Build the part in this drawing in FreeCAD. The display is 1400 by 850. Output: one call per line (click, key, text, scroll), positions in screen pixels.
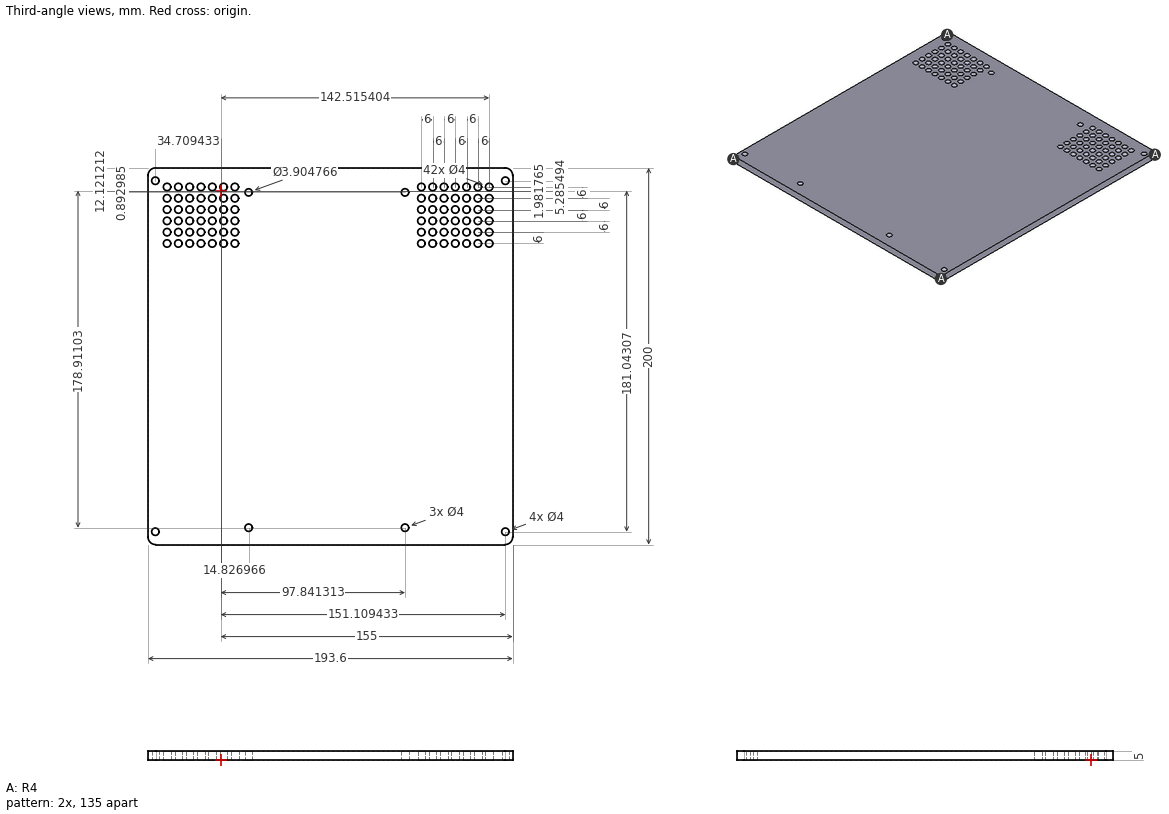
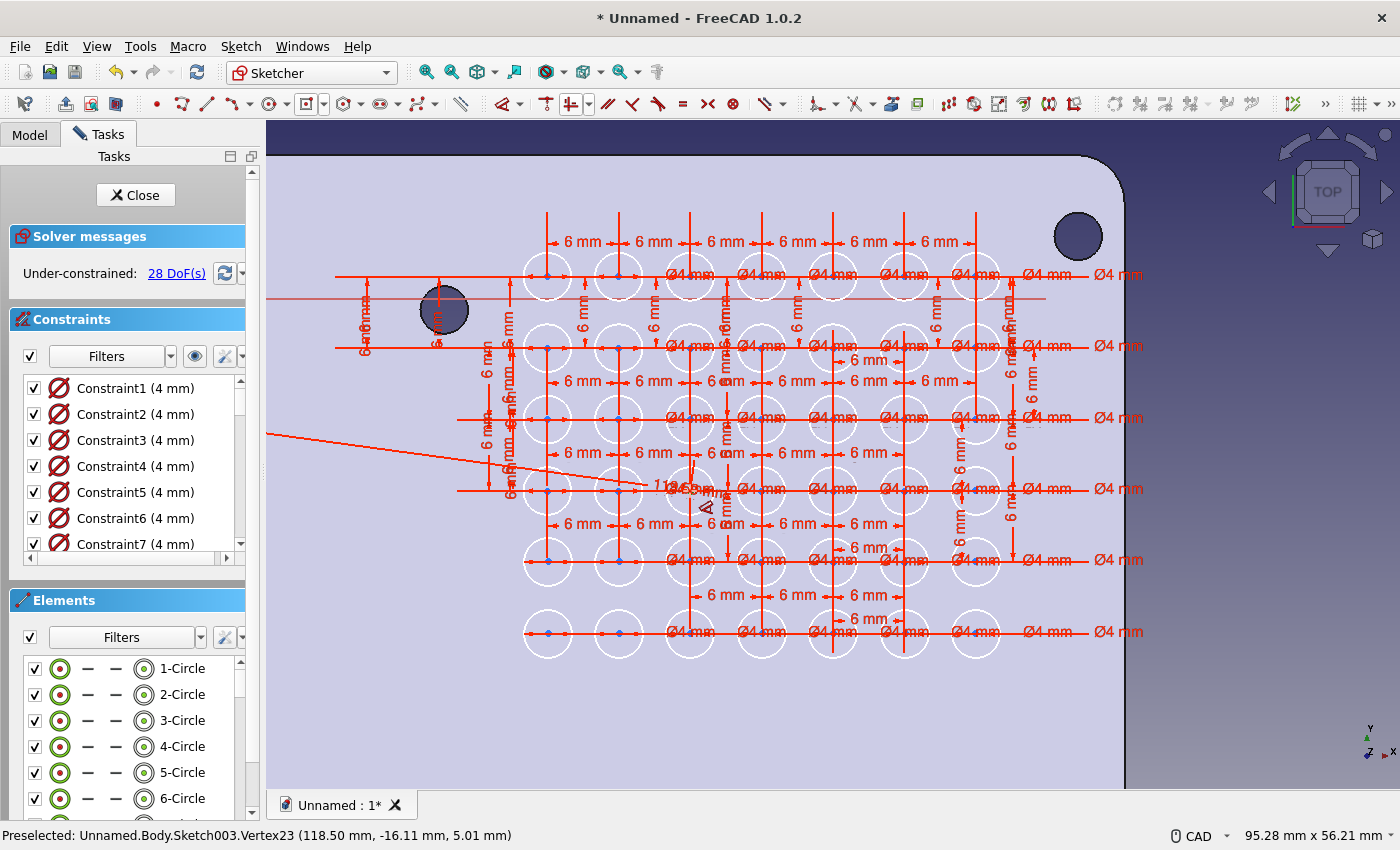
click(690, 562)
click(510, 527)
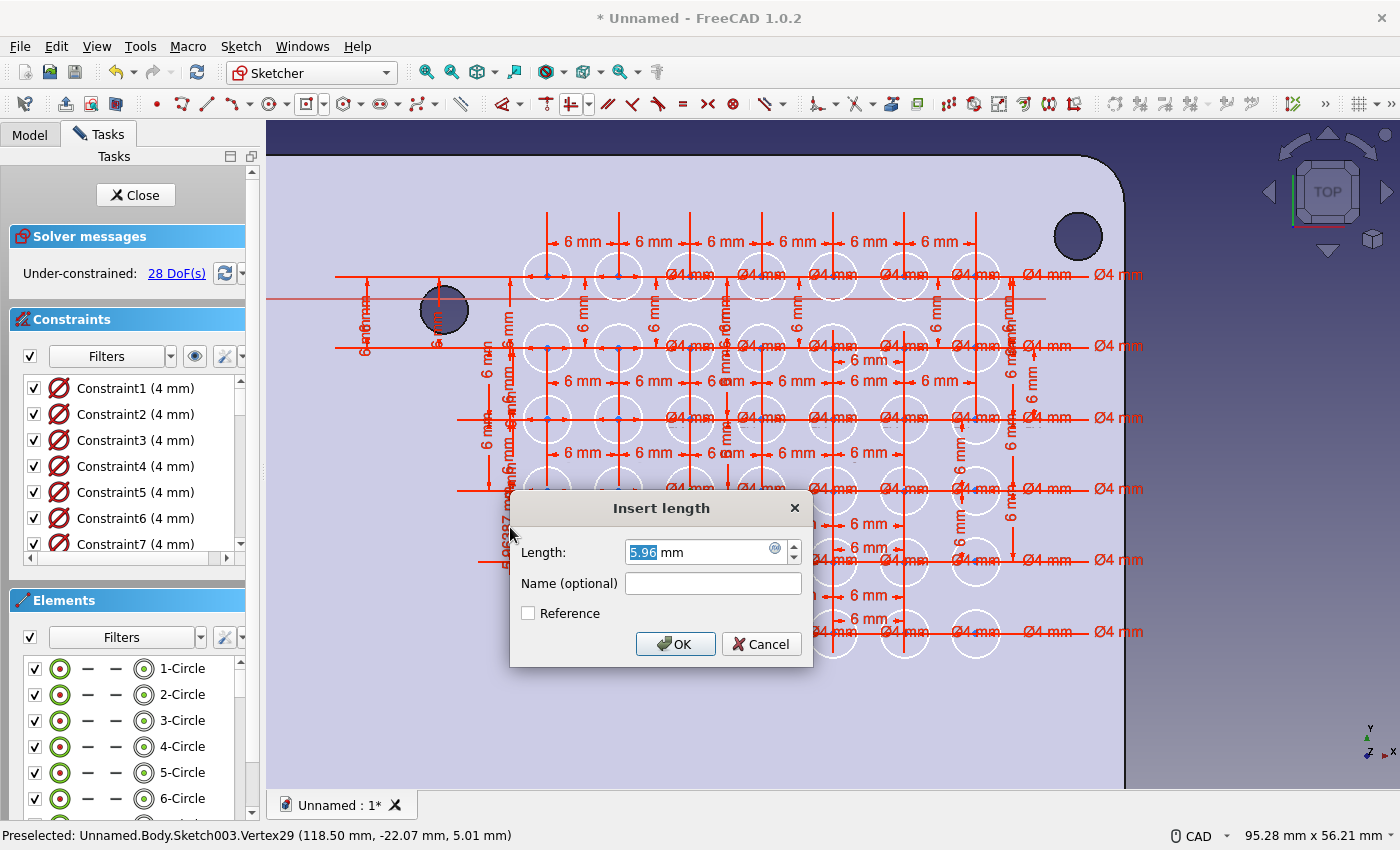
text(6)
key(Return)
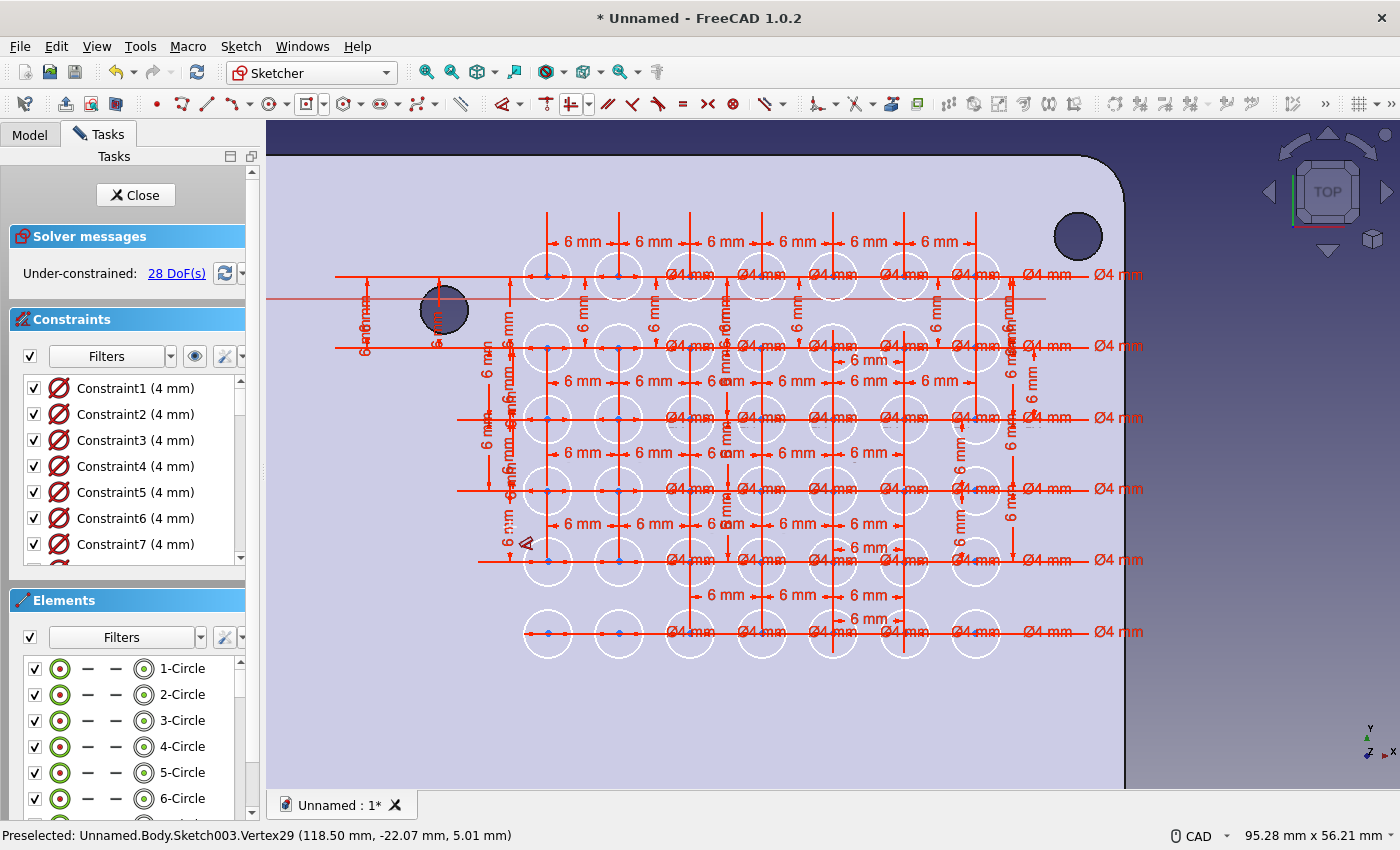
click(690, 562)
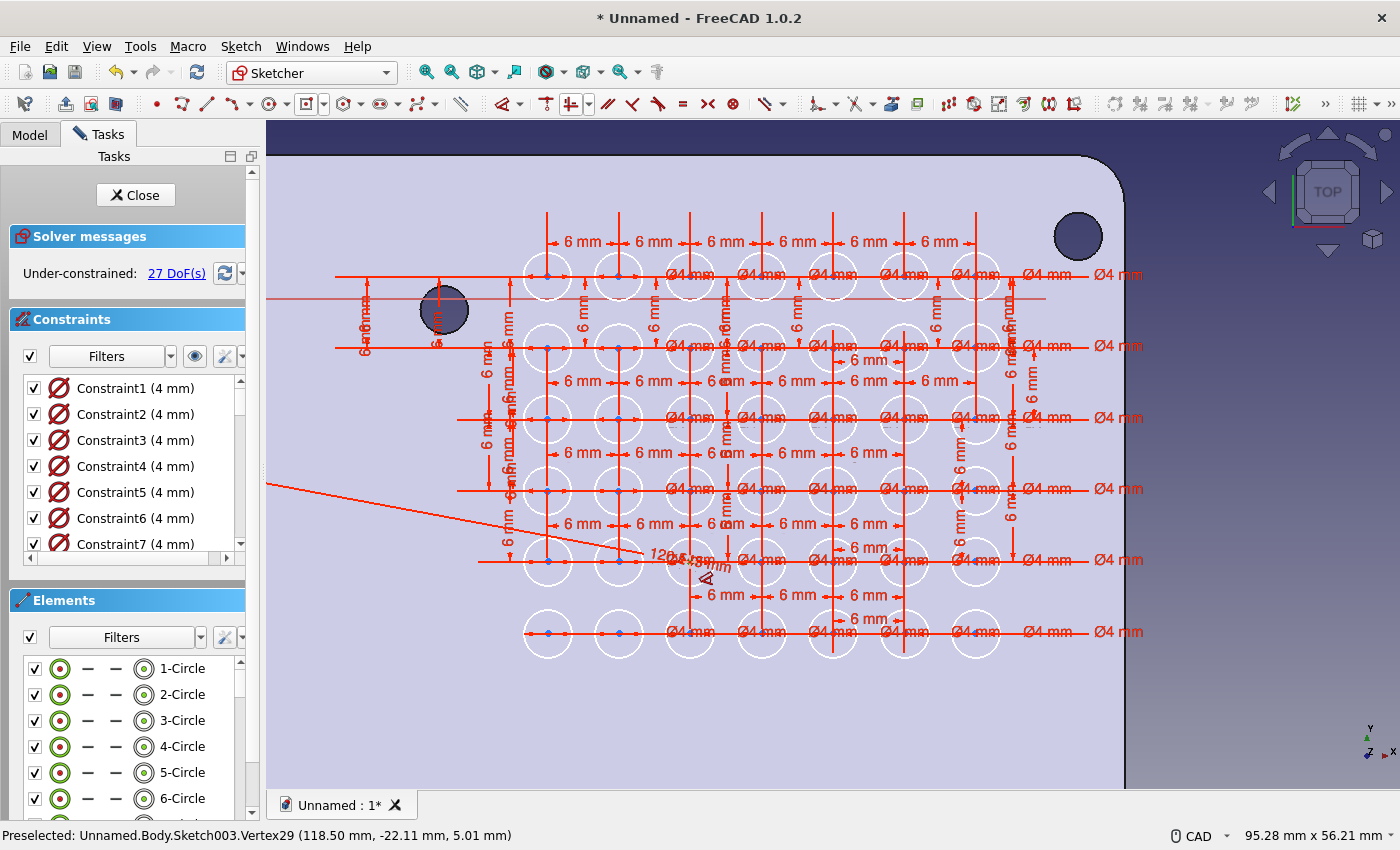
click(619, 562)
click(655, 596)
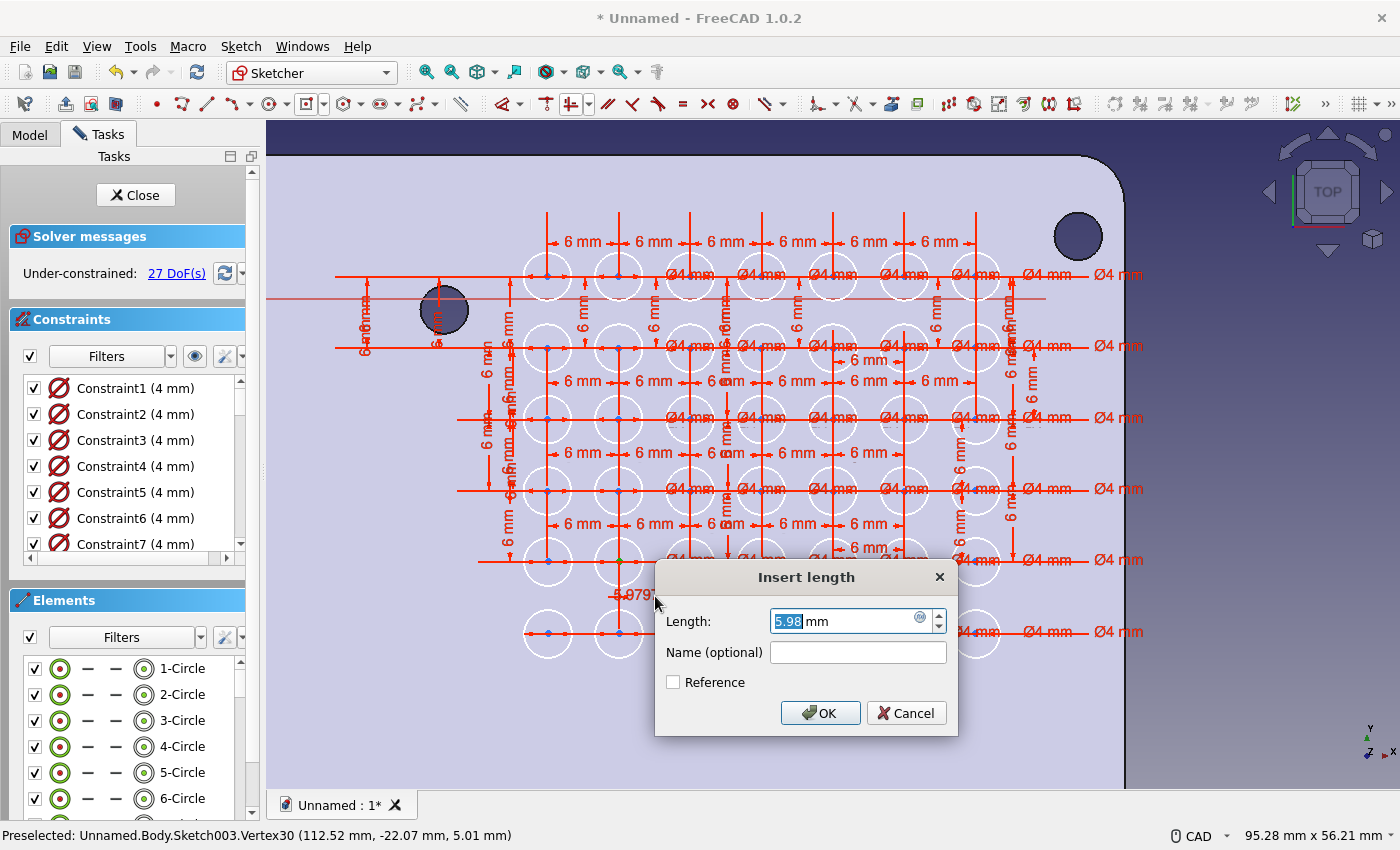
text(6)
key(Return)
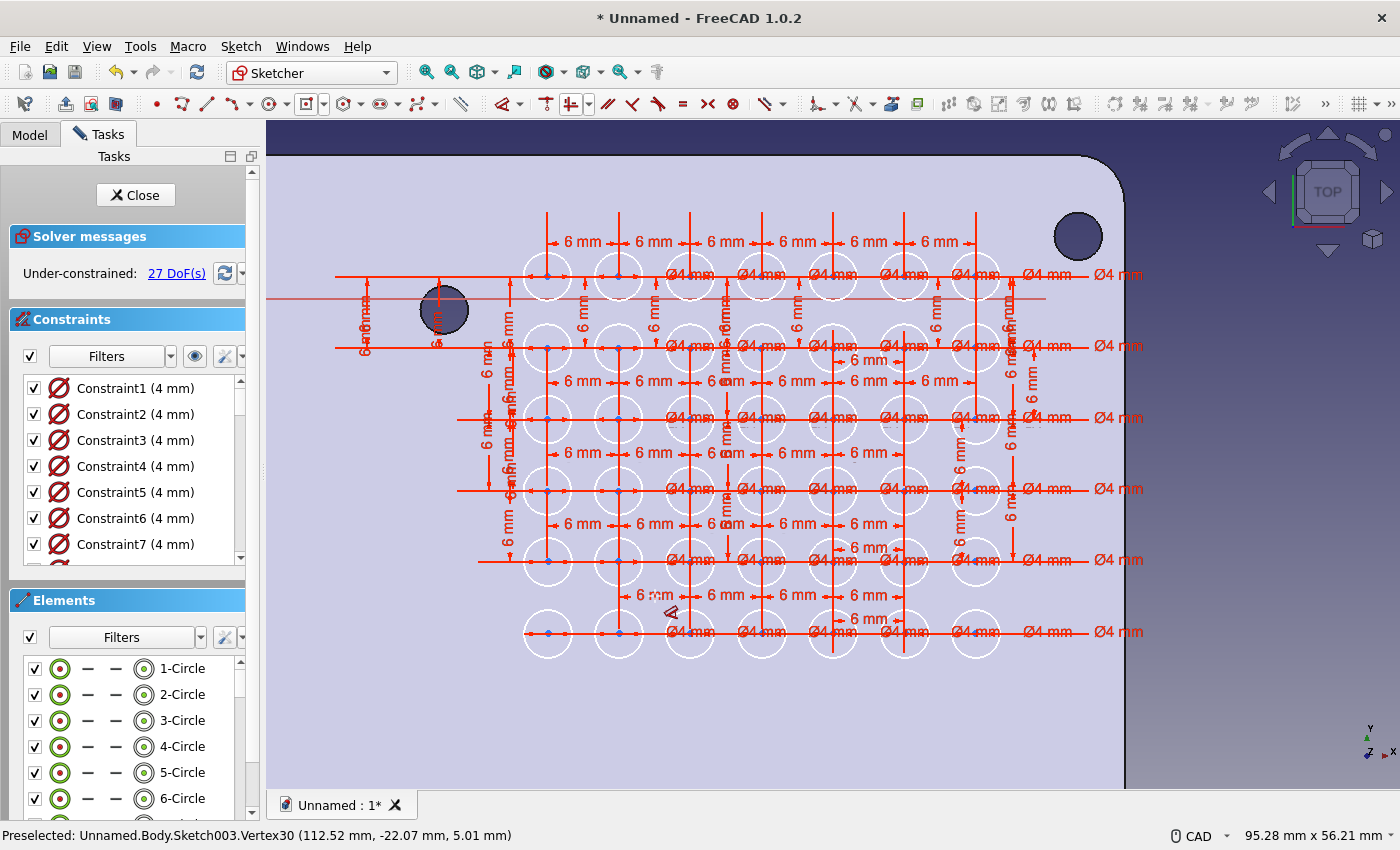
click(619, 491)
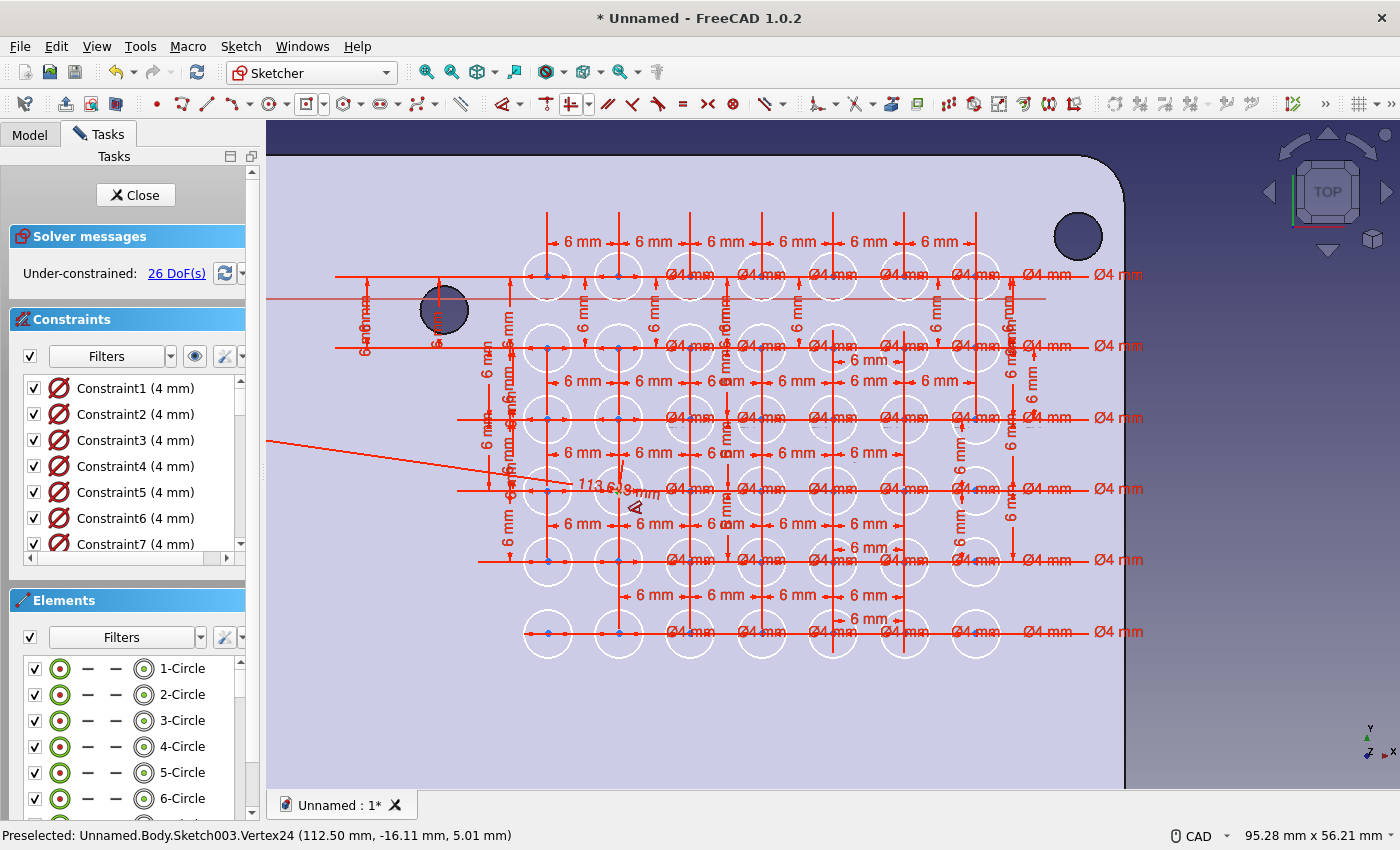
click(619, 562)
click(513, 551)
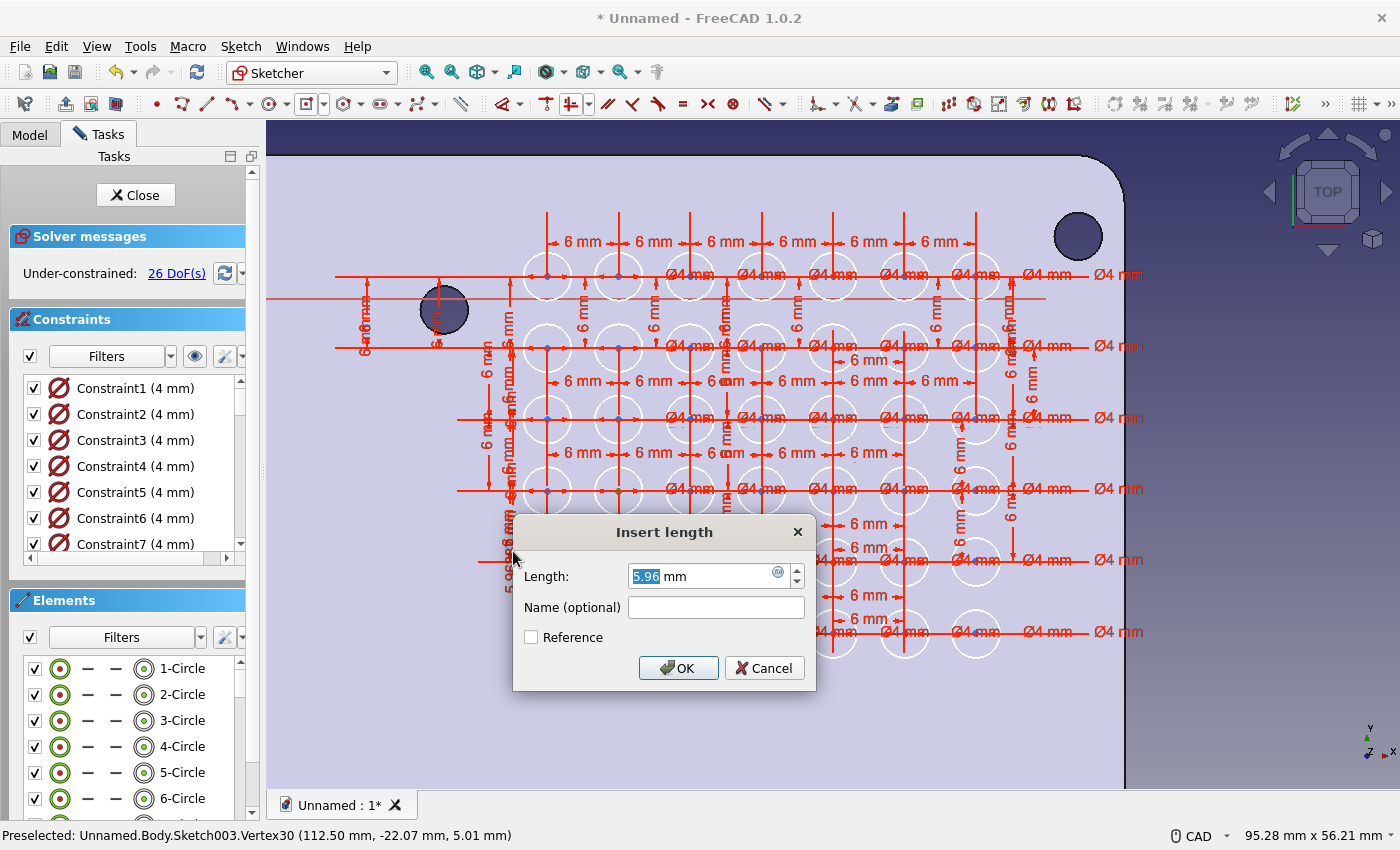
text(6)
key(Return)